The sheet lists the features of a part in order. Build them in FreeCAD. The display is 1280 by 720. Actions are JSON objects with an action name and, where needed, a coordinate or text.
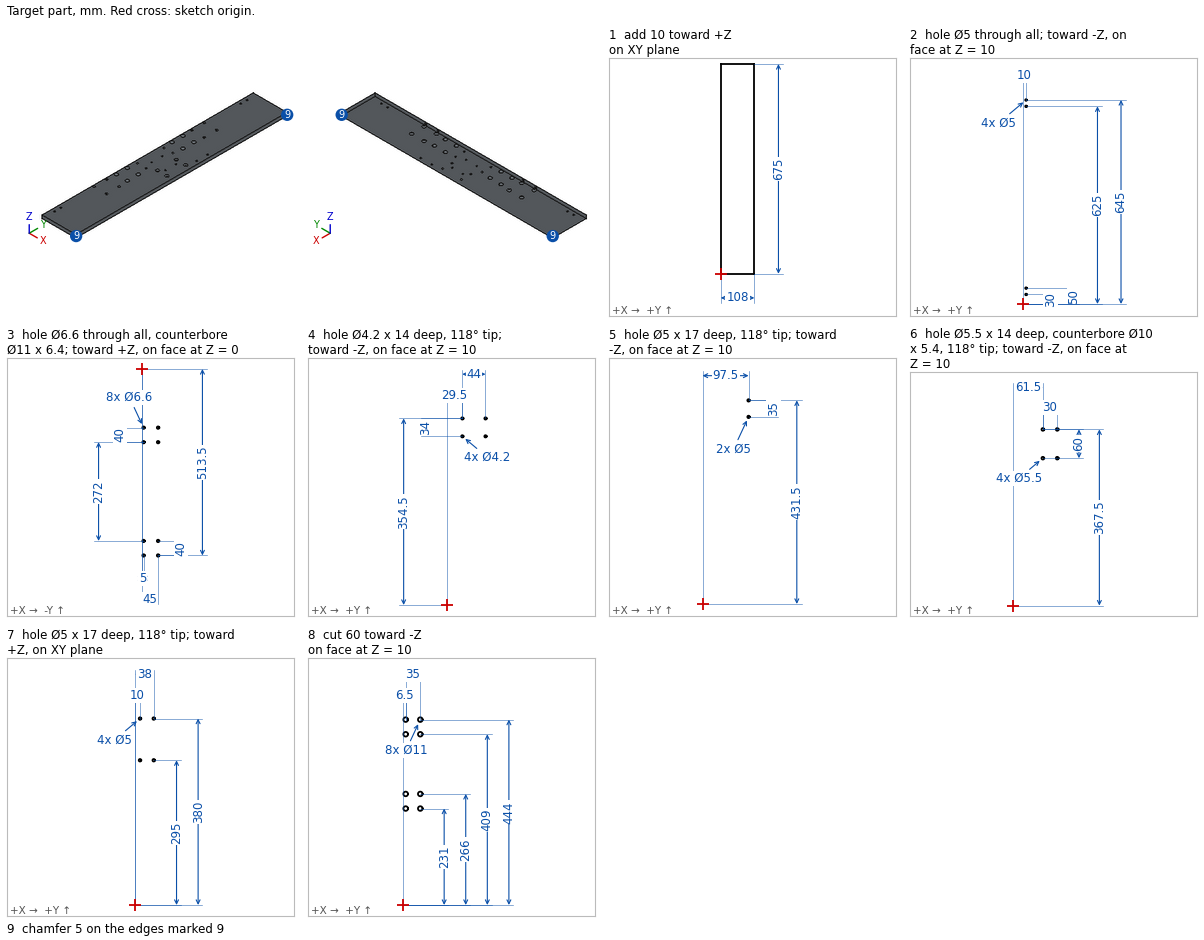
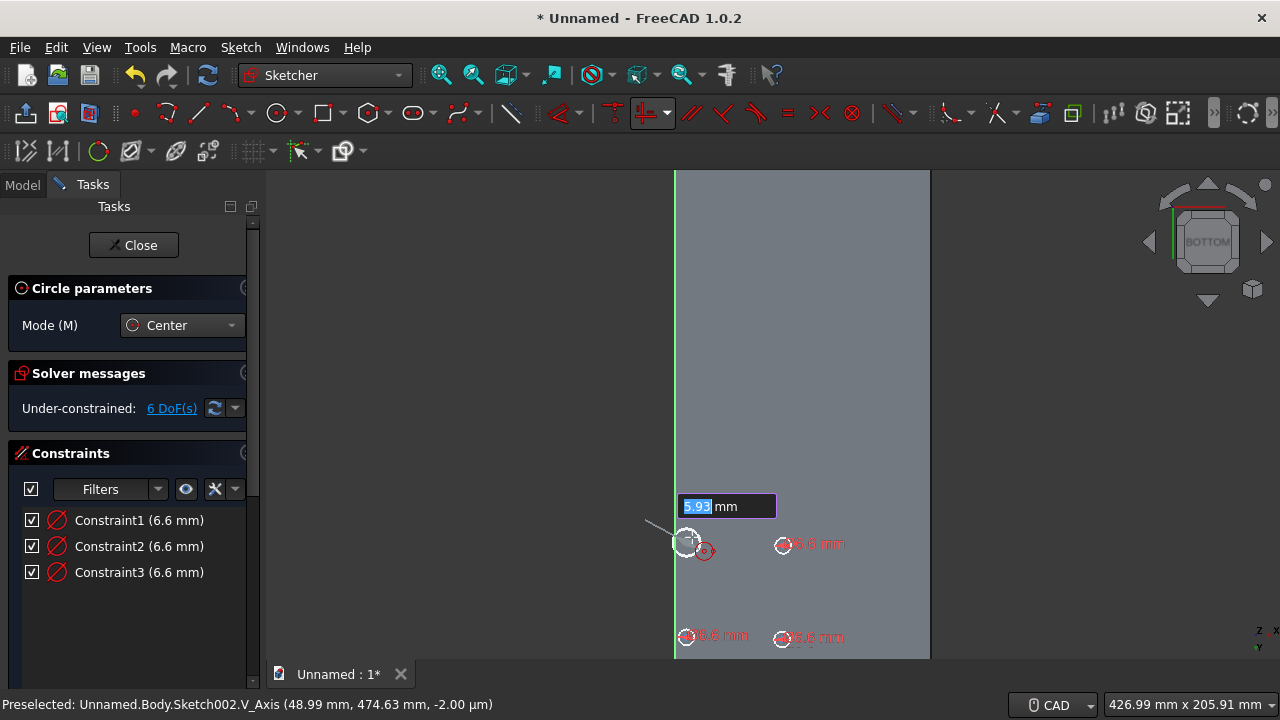
{"action": "type", "text": "6.6"}
{"action": "key", "text": "Return"}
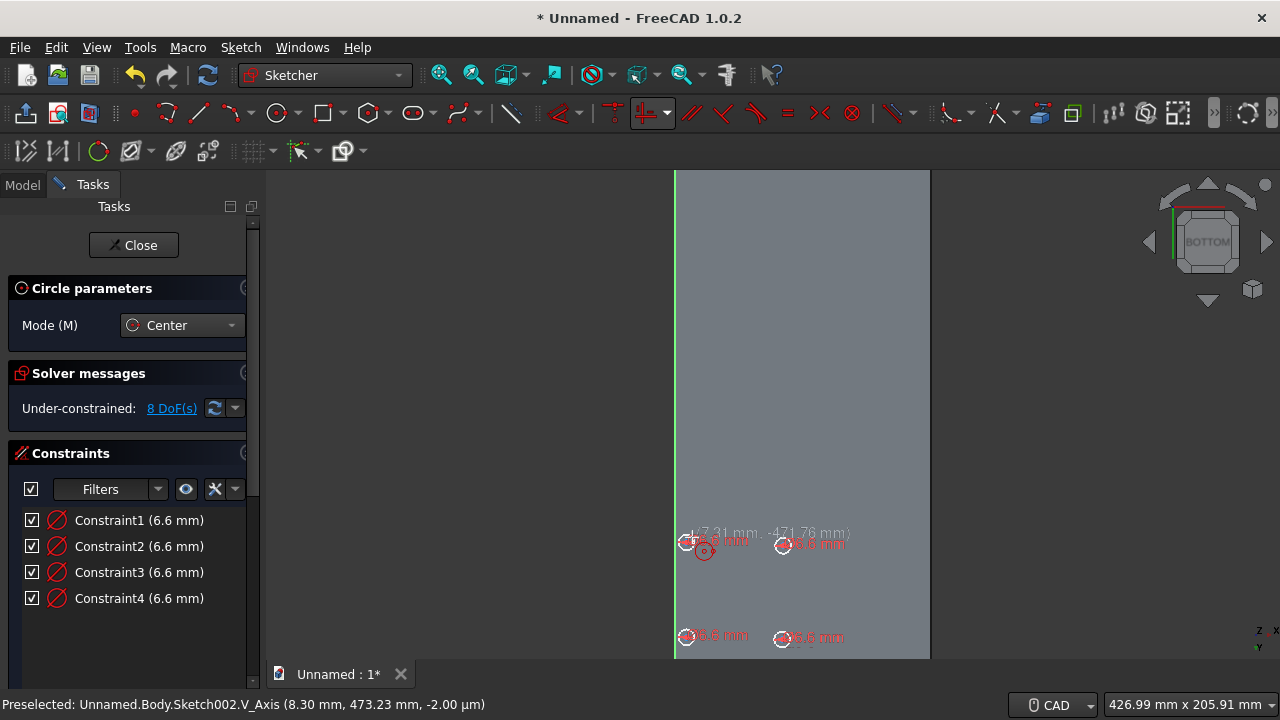
{"action": "scroll", "coordinate": [695, 540], "scroll_direction": "down", "scroll_amount": 7}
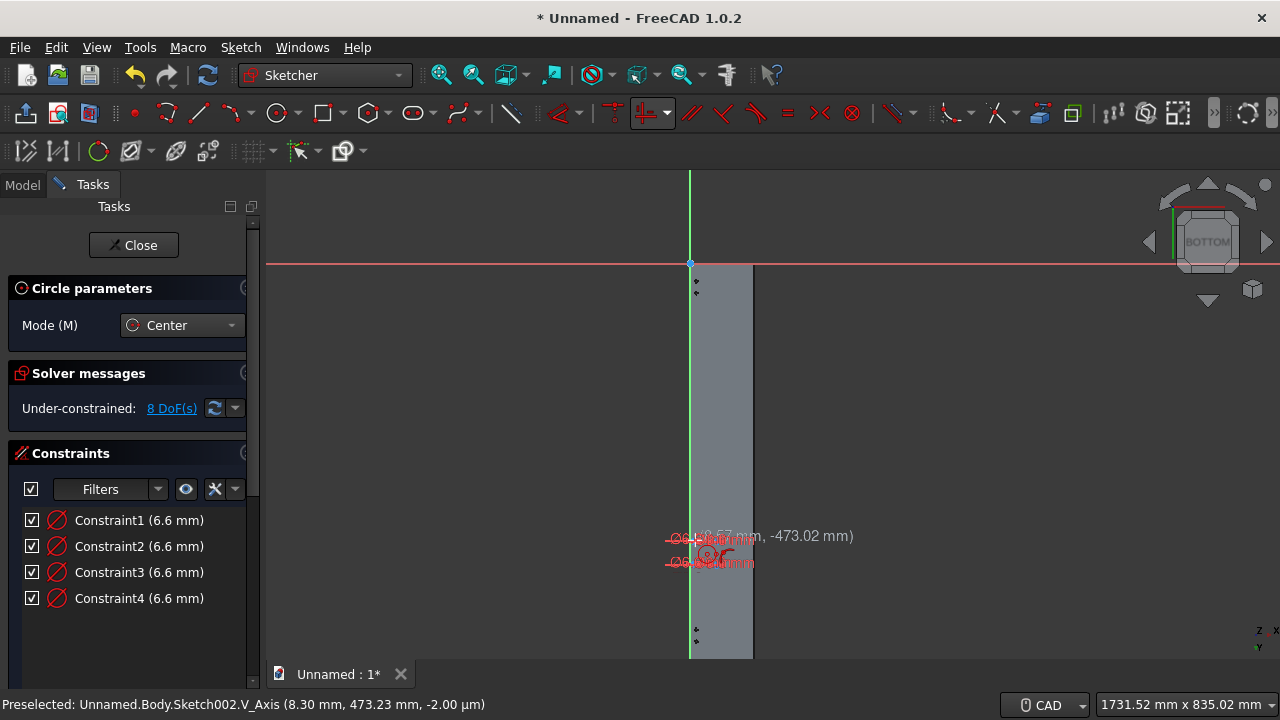
{"action": "scroll", "coordinate": [693, 382], "scroll_direction": "up", "scroll_amount": 13}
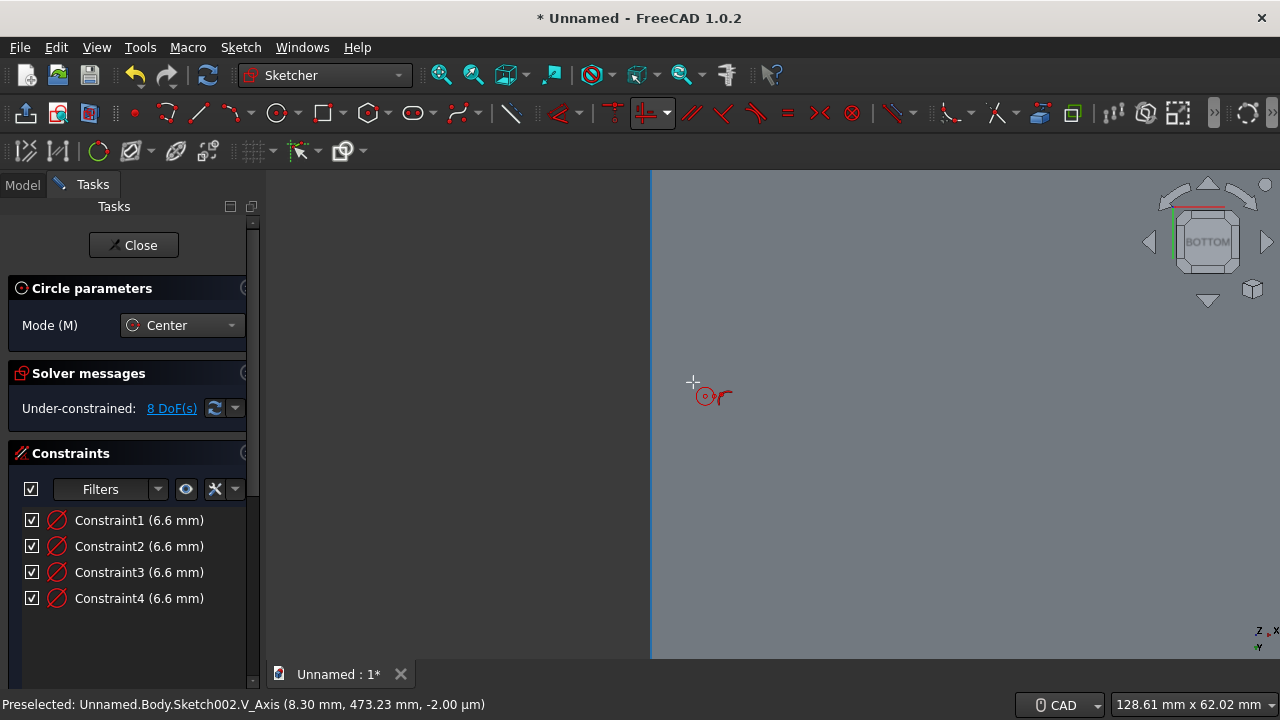
{"action": "left_click", "coordinate": [691, 374]}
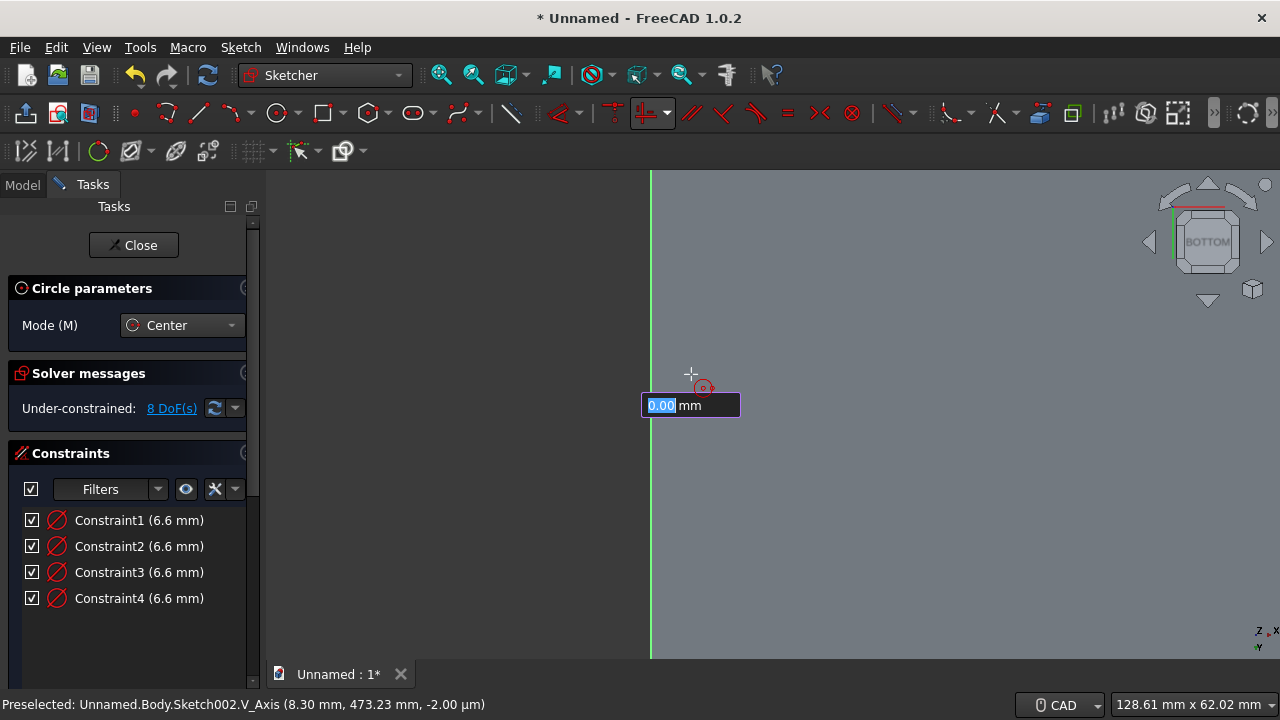
{"action": "scroll", "coordinate": [693, 382], "scroll_direction": "down", "scroll_amount": 13}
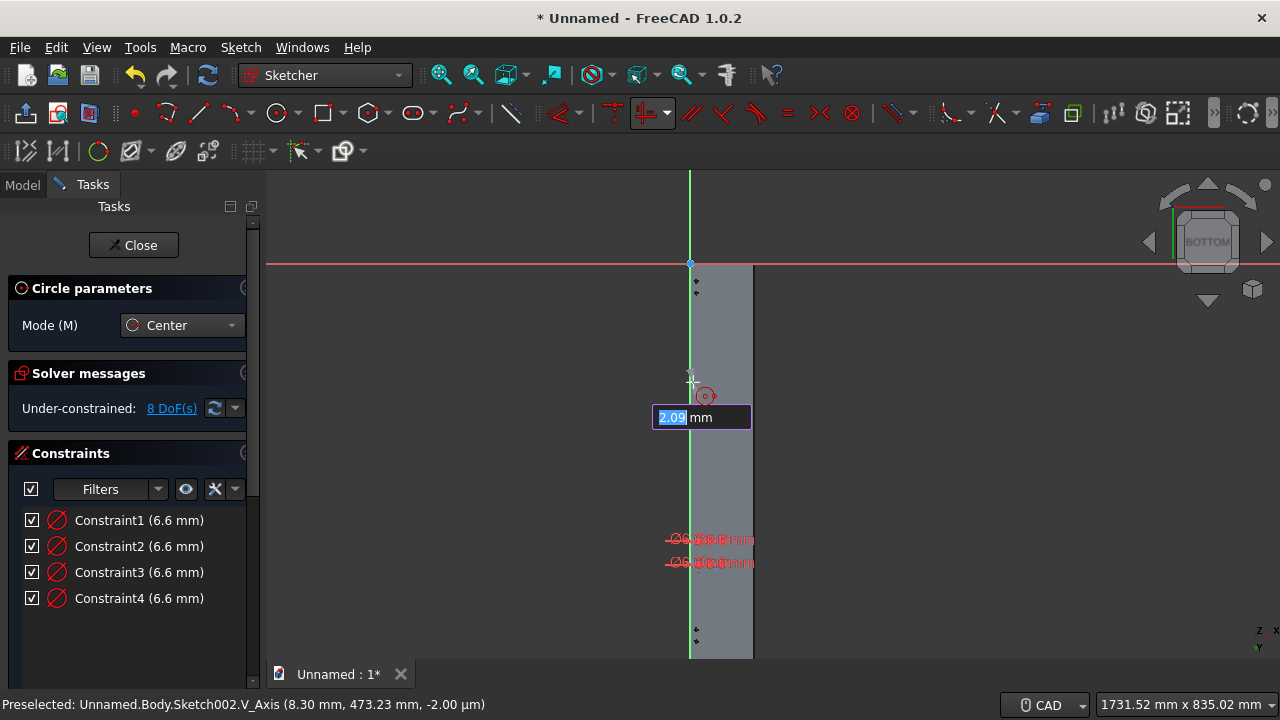
{"action": "scroll", "coordinate": [695, 380], "scroll_direction": "up", "scroll_amount": 7}
{"action": "mouse_move", "coordinate": [692, 380]}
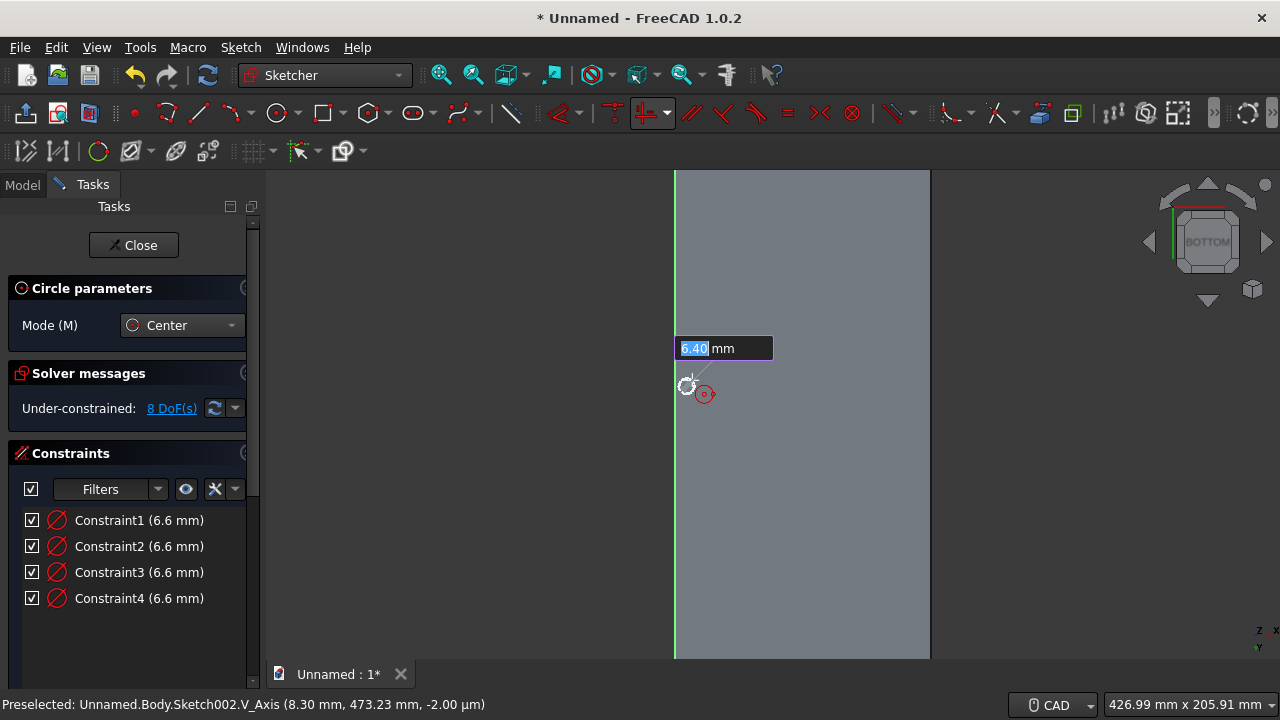
{"action": "type", "text": "6.6"}
{"action": "key", "text": "Return"}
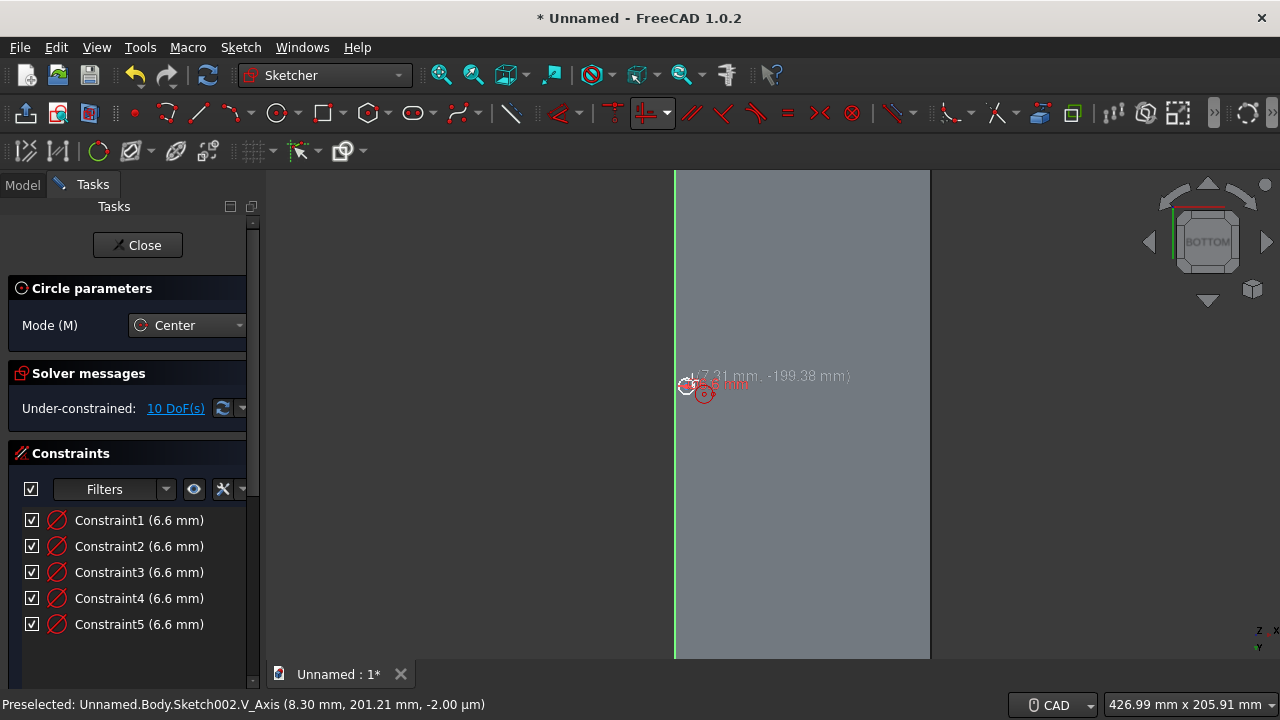
{"action": "scroll", "coordinate": [782, 386], "scroll_direction": "up", "scroll_amount": 6}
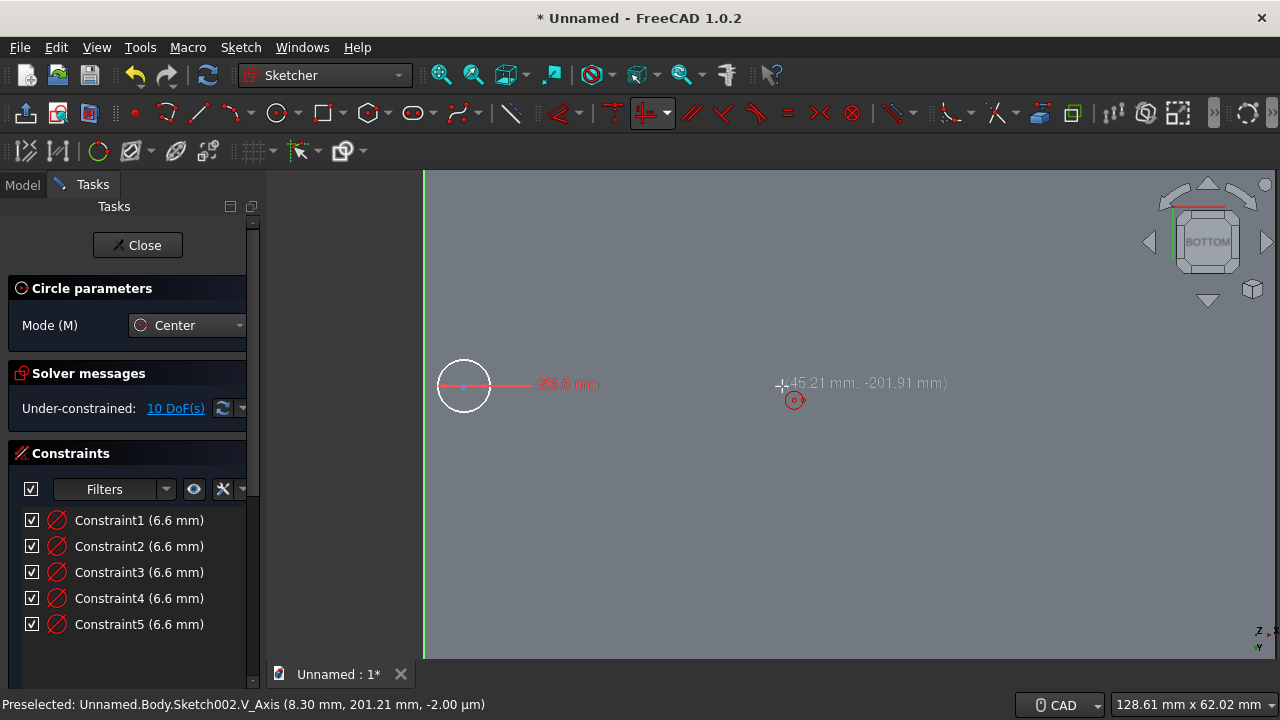
{"action": "scroll", "coordinate": [712, 381], "scroll_direction": "down", "scroll_amount": 13}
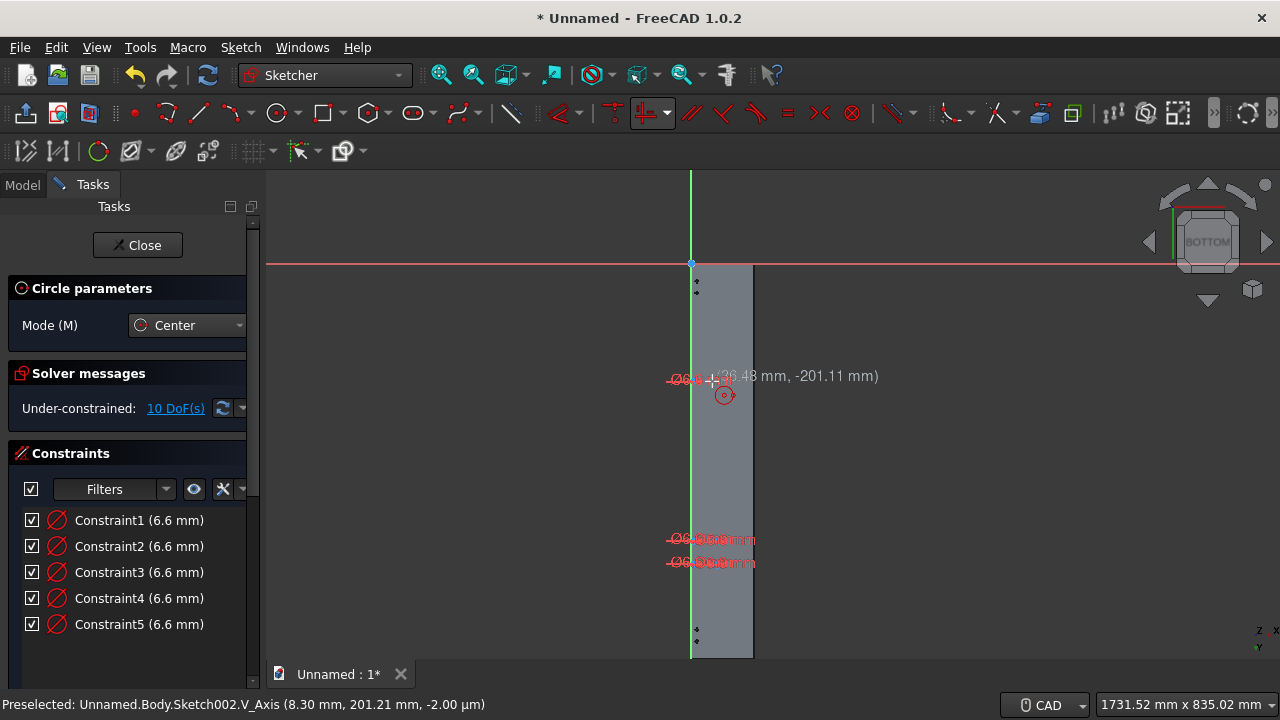
{"action": "left_click", "coordinate": [717, 382]}
{"action": "mouse_move", "coordinate": [719, 380]}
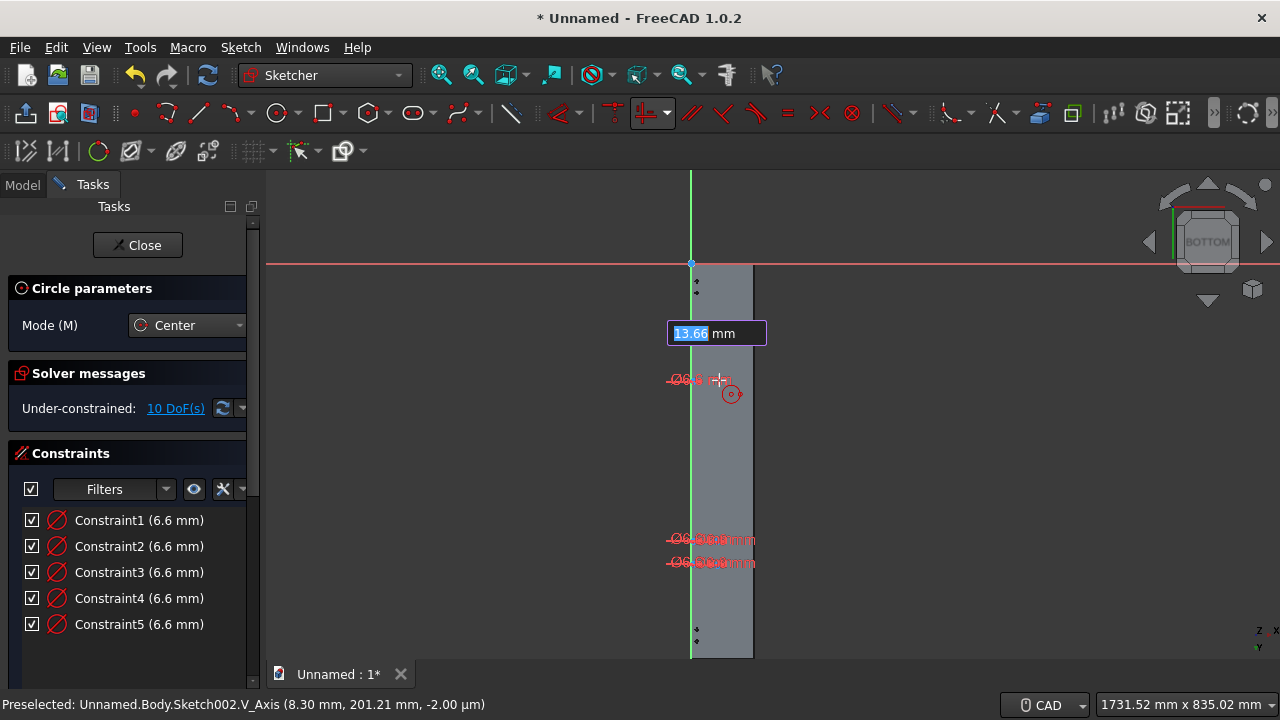
{"action": "type", "text": "6.6"}
{"action": "key", "text": "Return"}